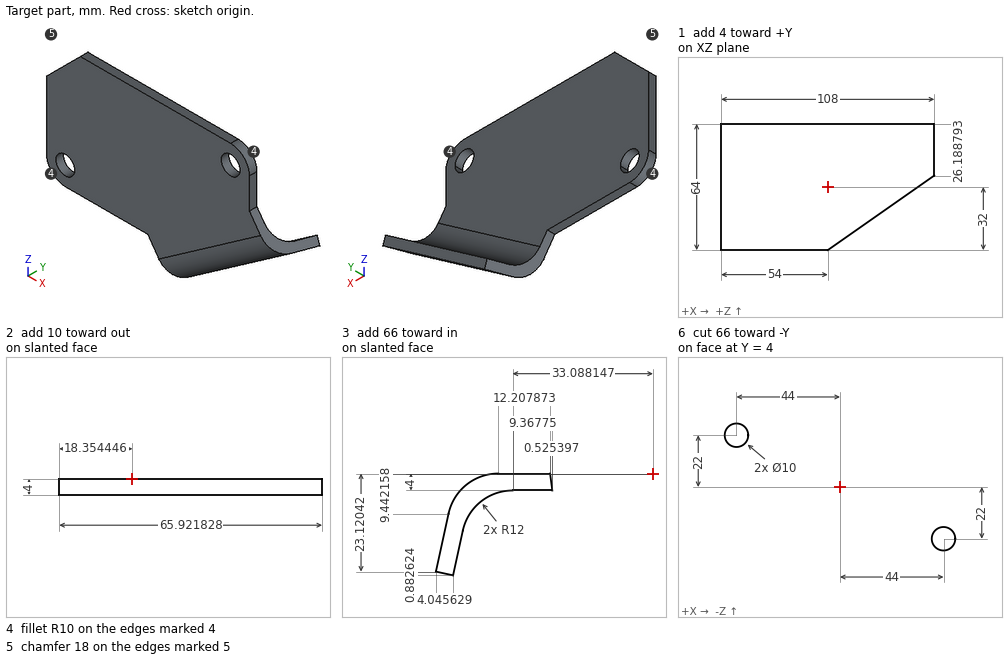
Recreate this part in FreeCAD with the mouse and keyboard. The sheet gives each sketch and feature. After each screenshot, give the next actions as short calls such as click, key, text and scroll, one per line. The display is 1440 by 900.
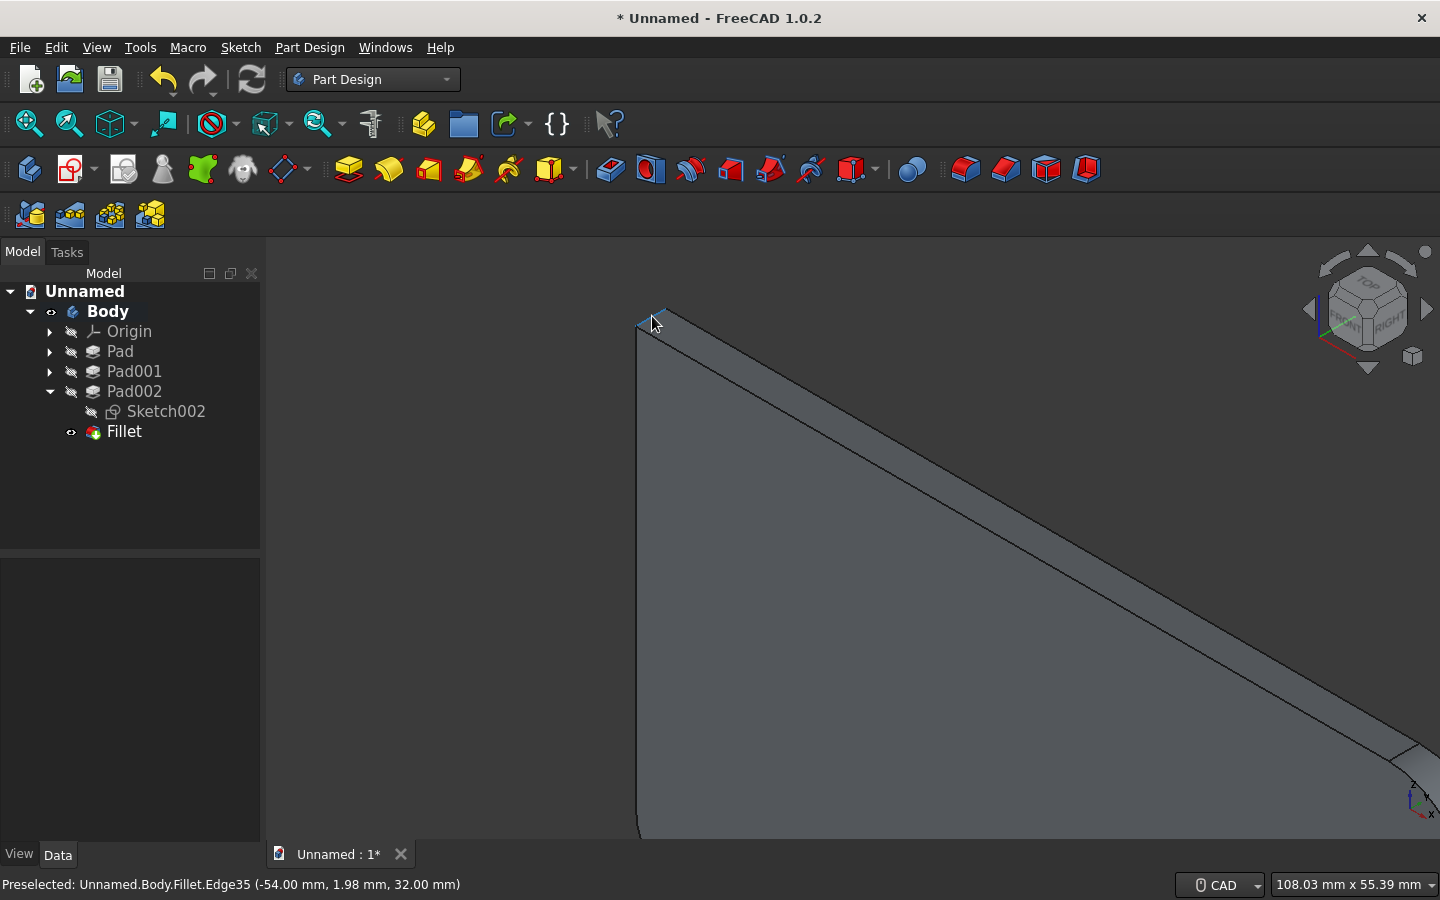
click(30, 124)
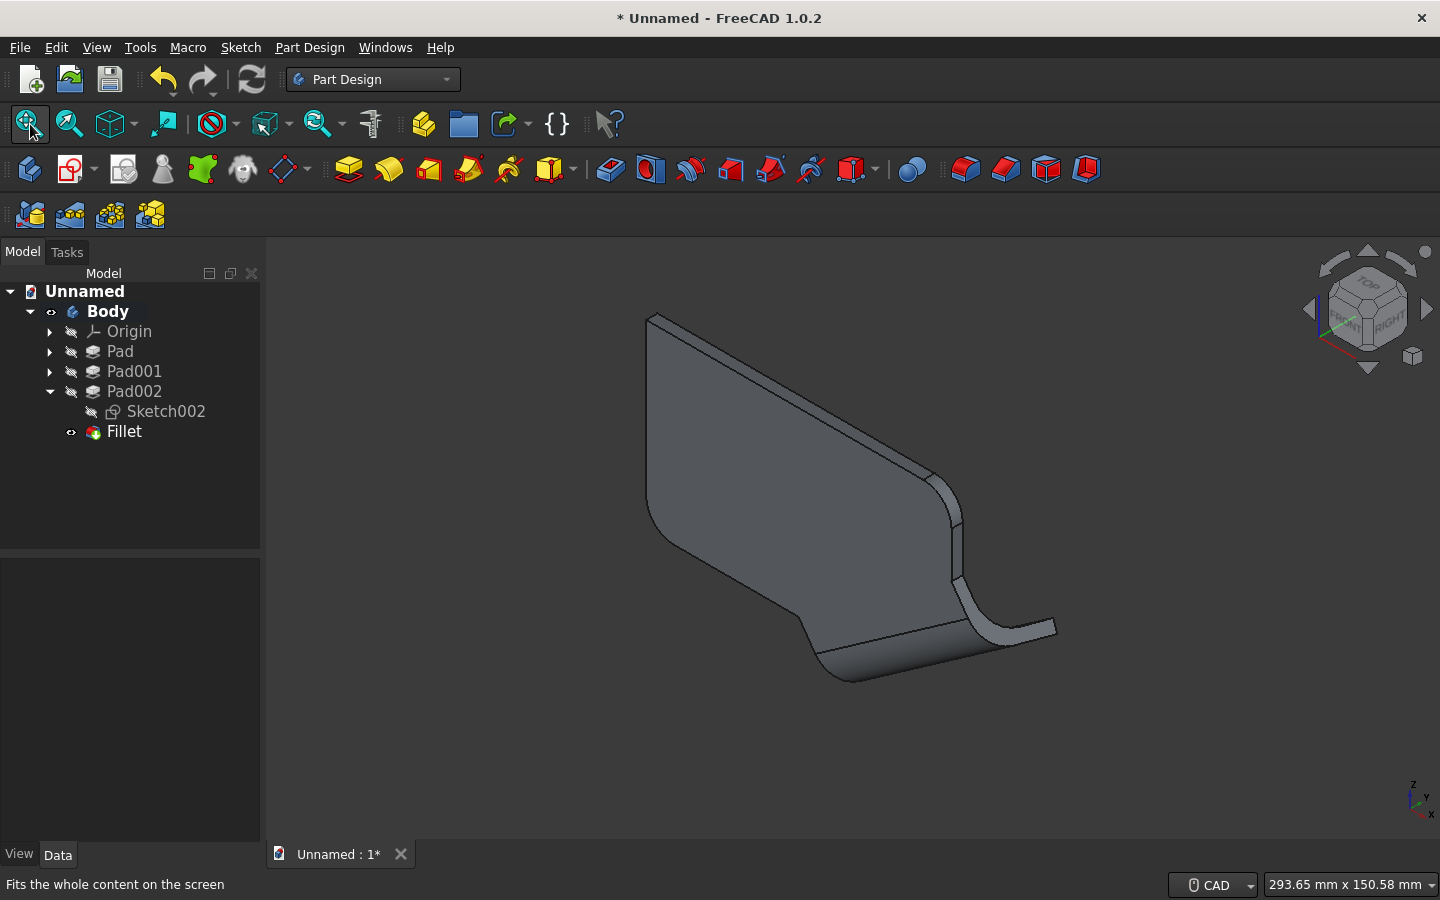
key(2)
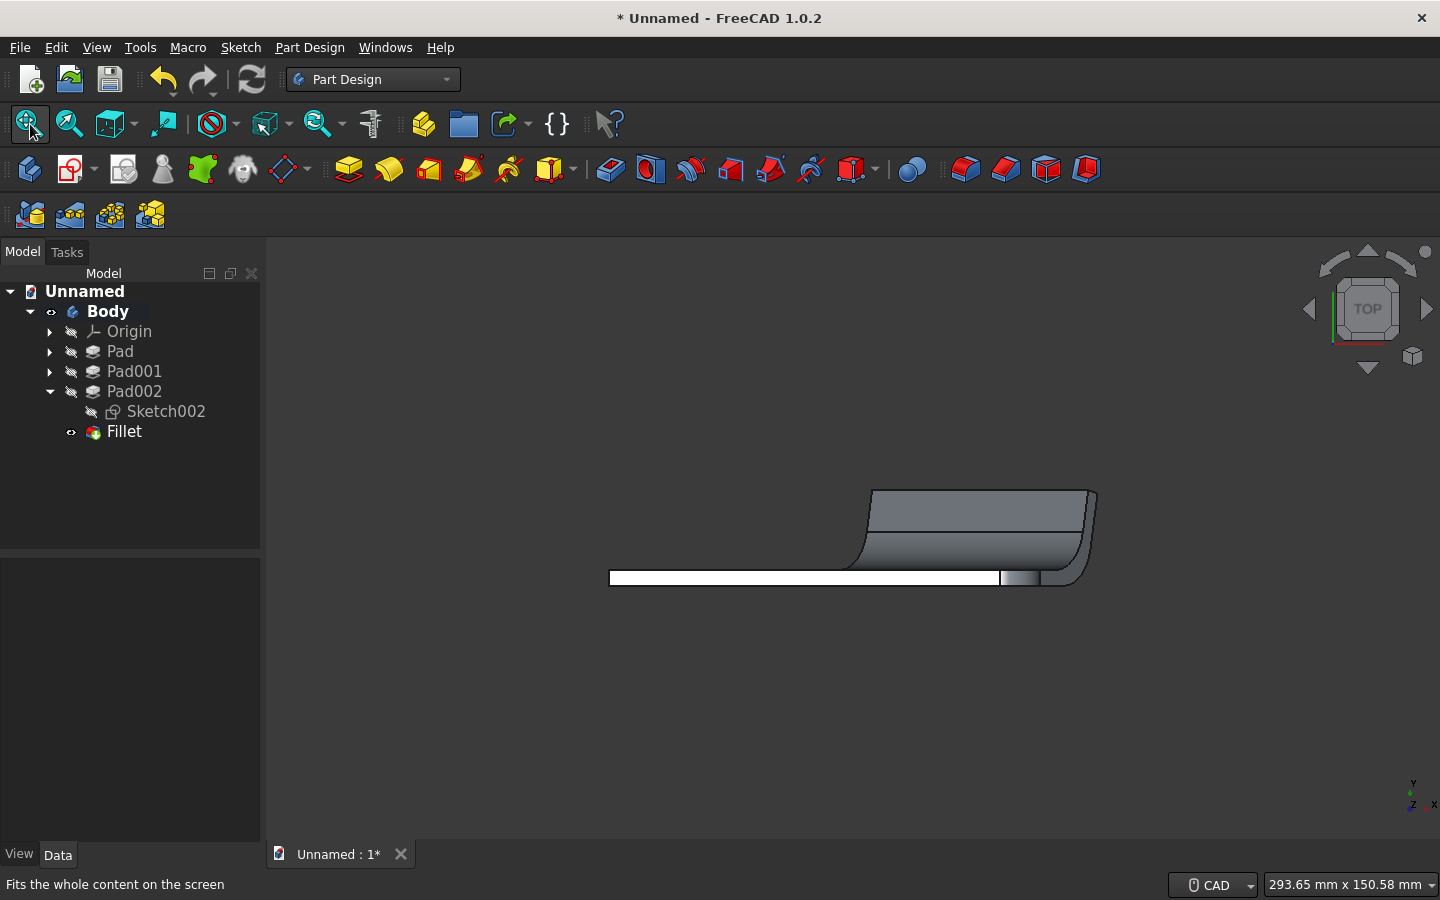
key(v)
key(f)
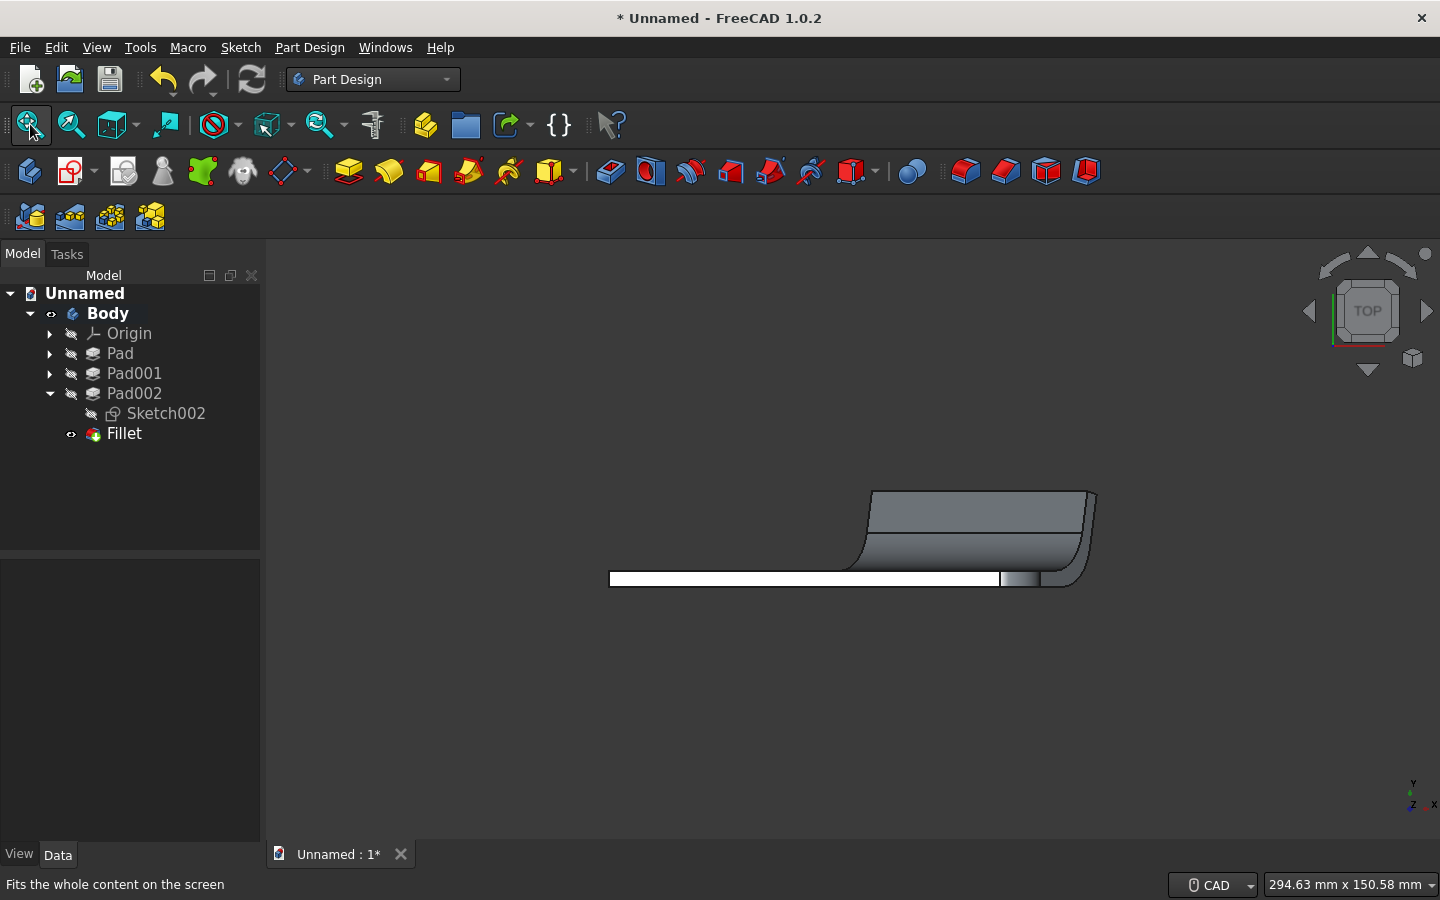
click(609, 578)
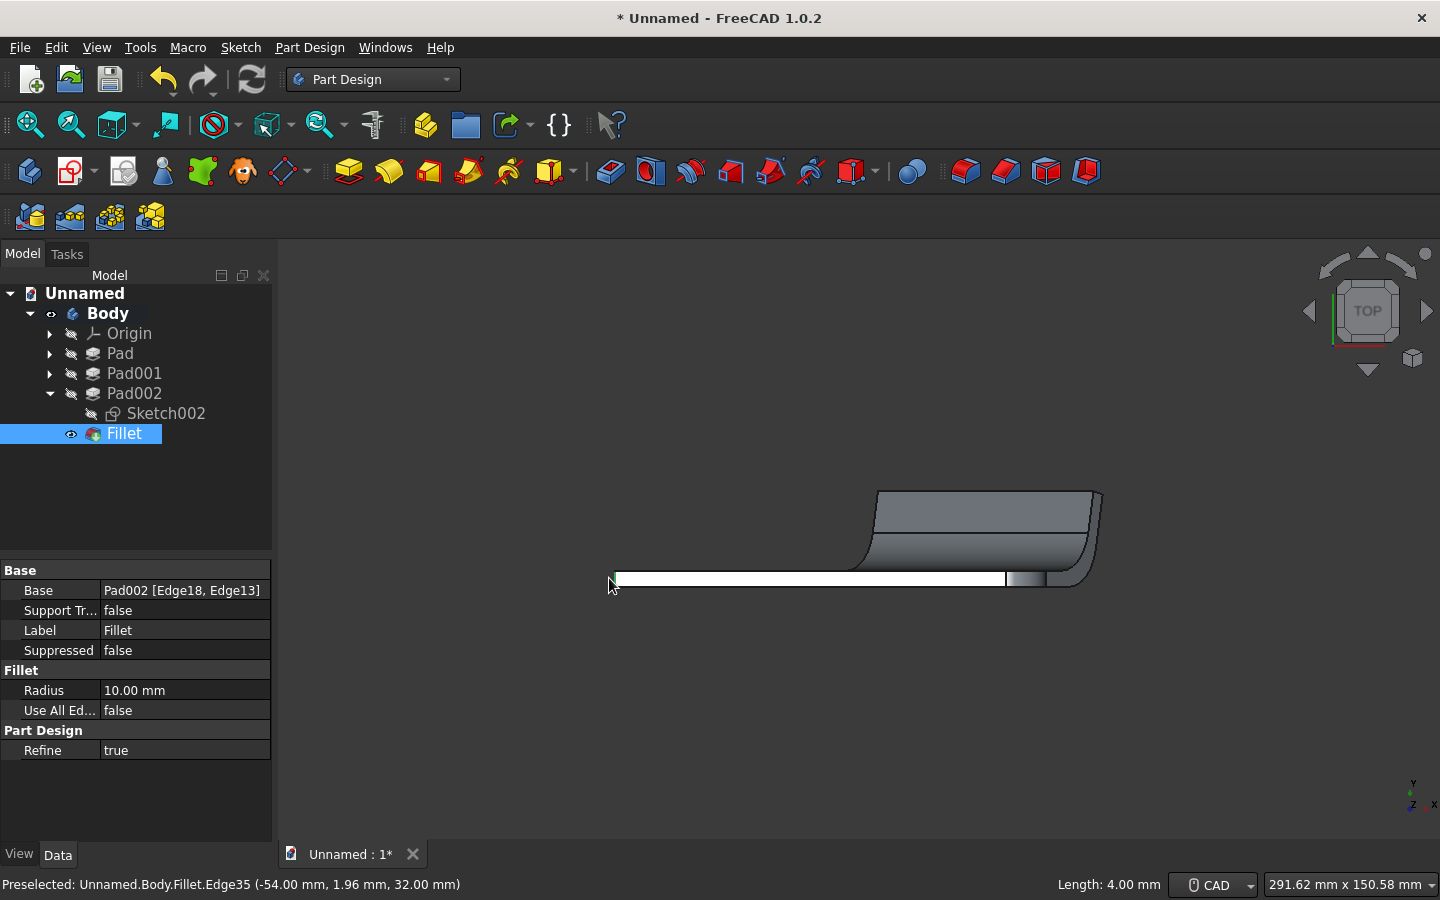
click(1006, 172)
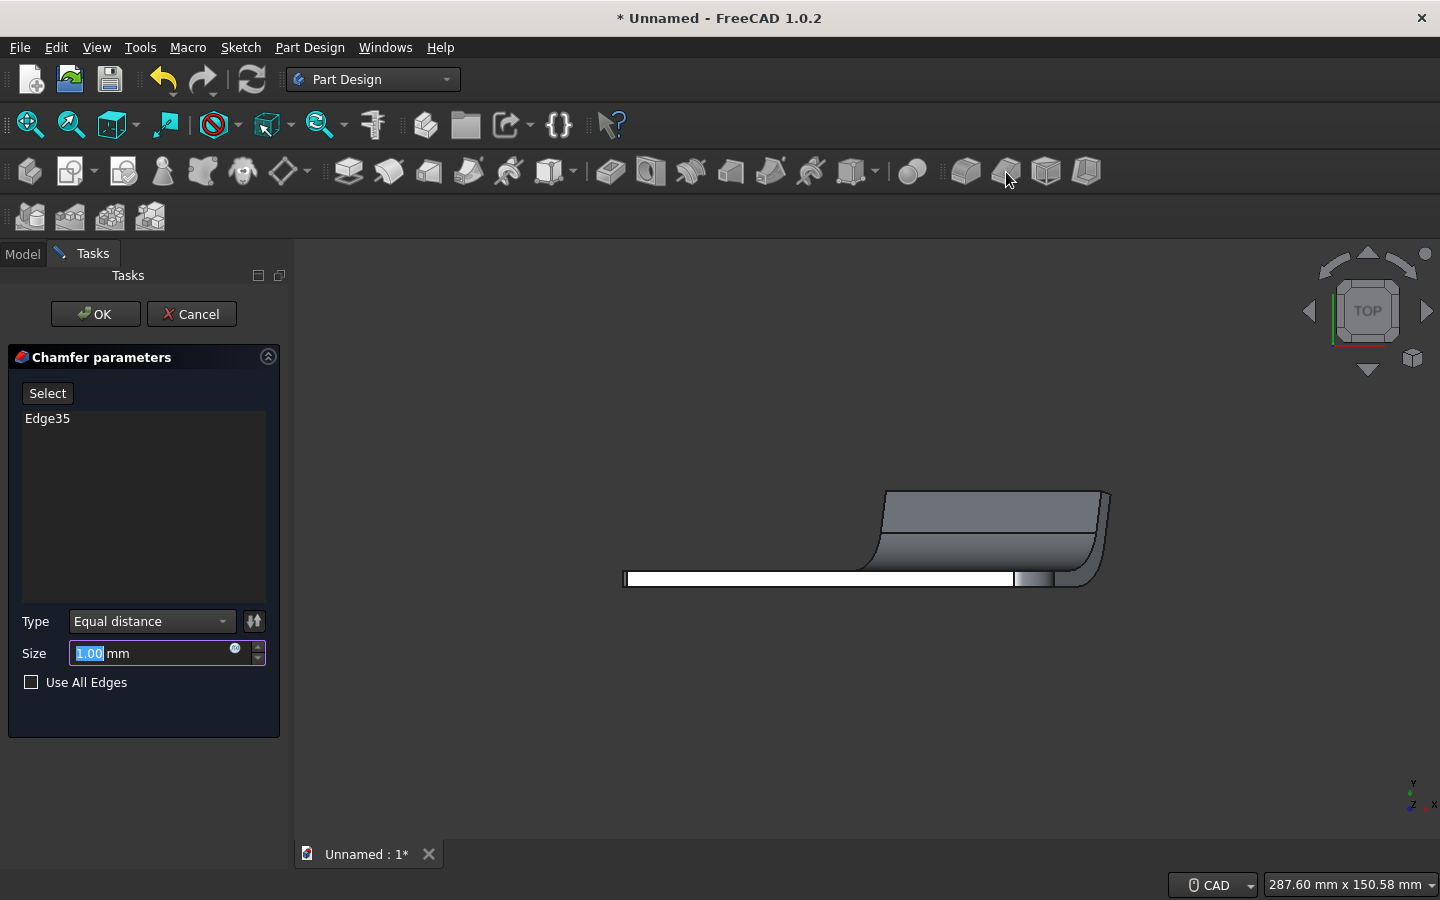
text(18)
key(Tab)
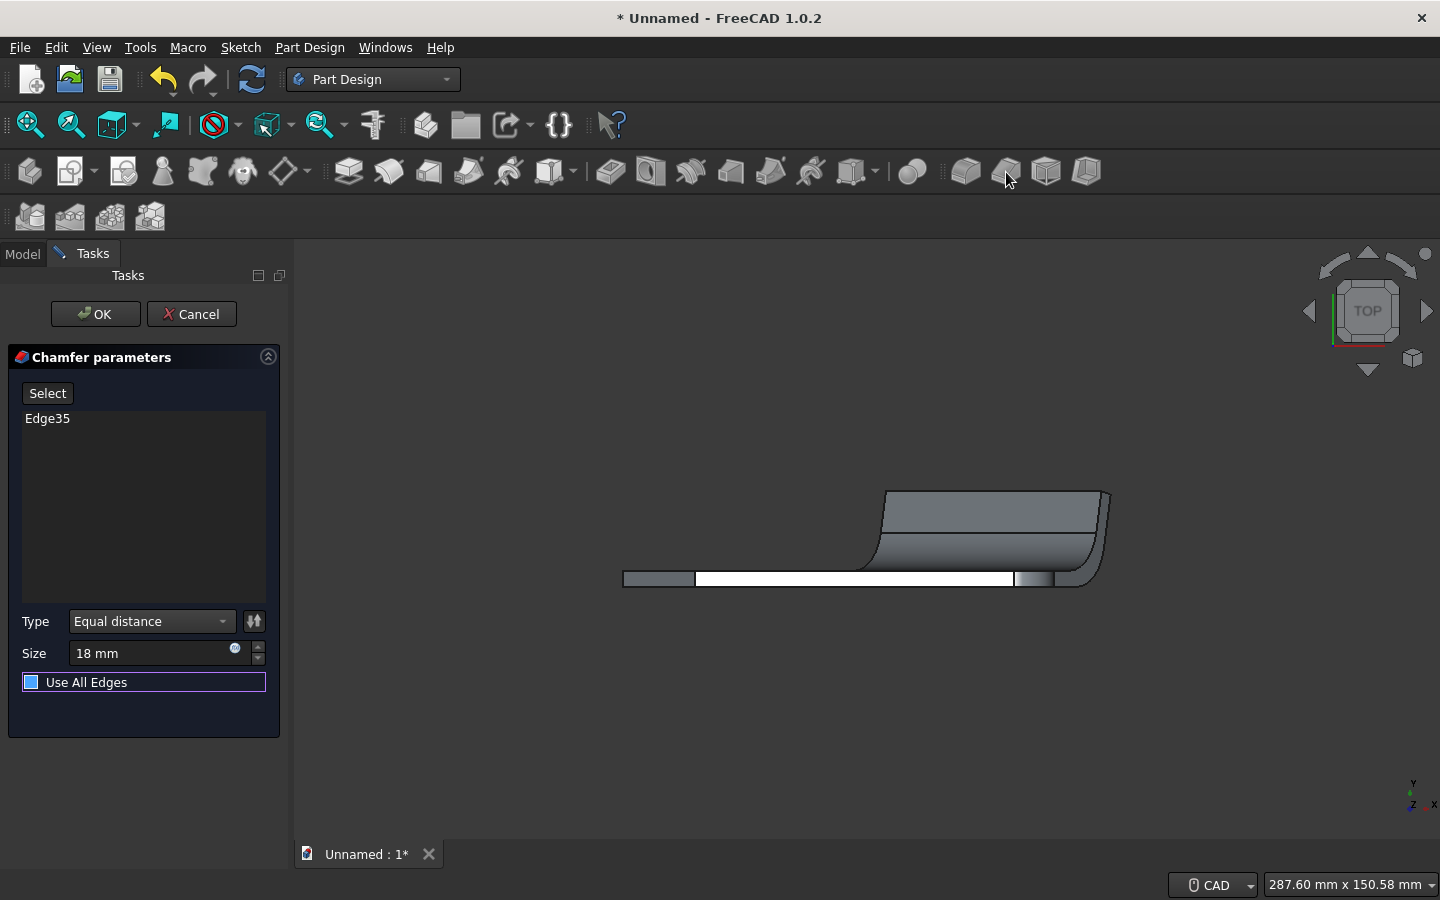
click(96, 314)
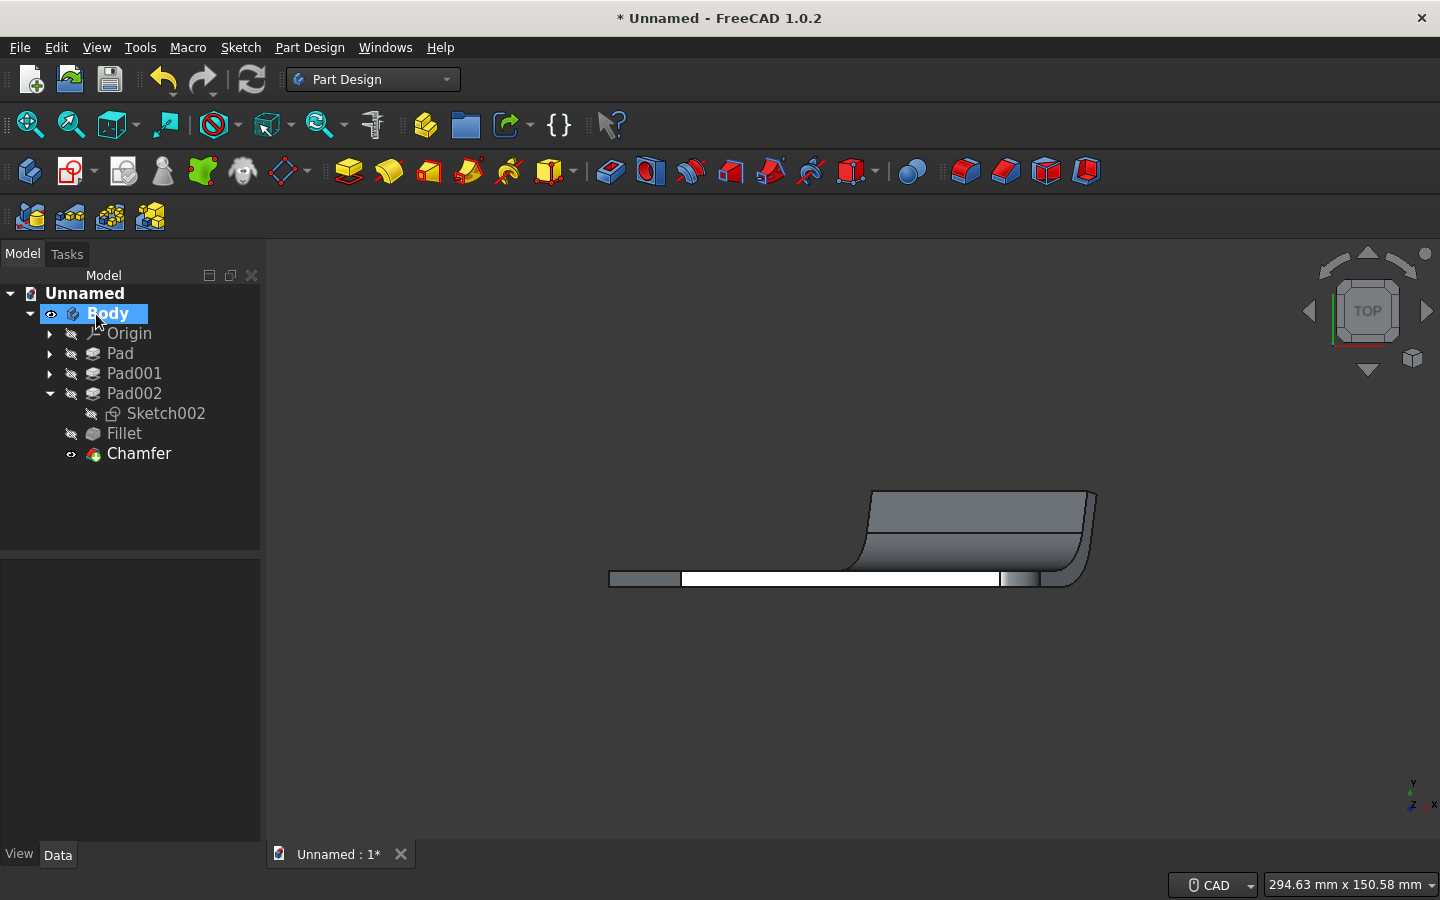
click(32, 126)